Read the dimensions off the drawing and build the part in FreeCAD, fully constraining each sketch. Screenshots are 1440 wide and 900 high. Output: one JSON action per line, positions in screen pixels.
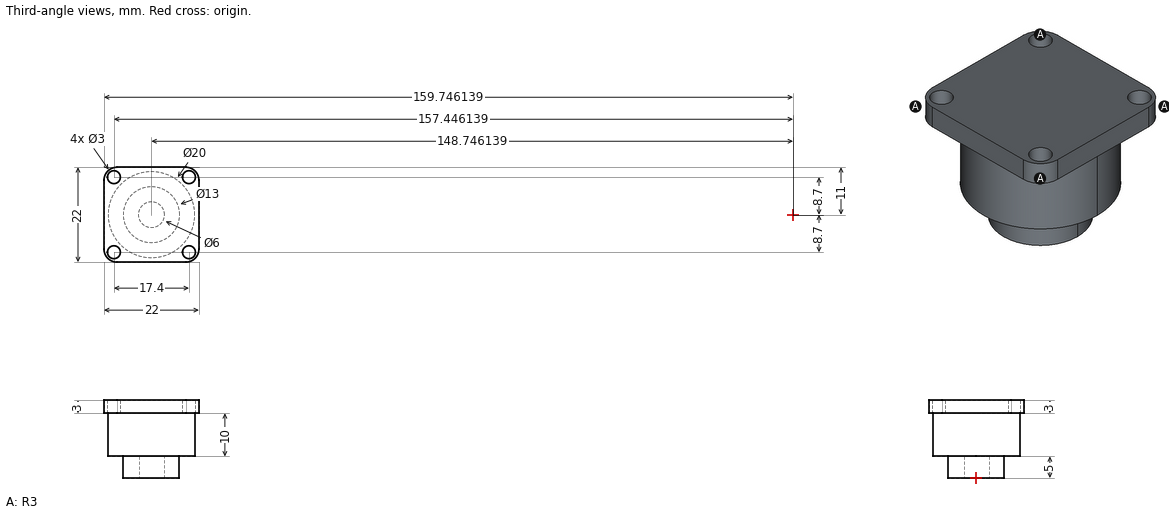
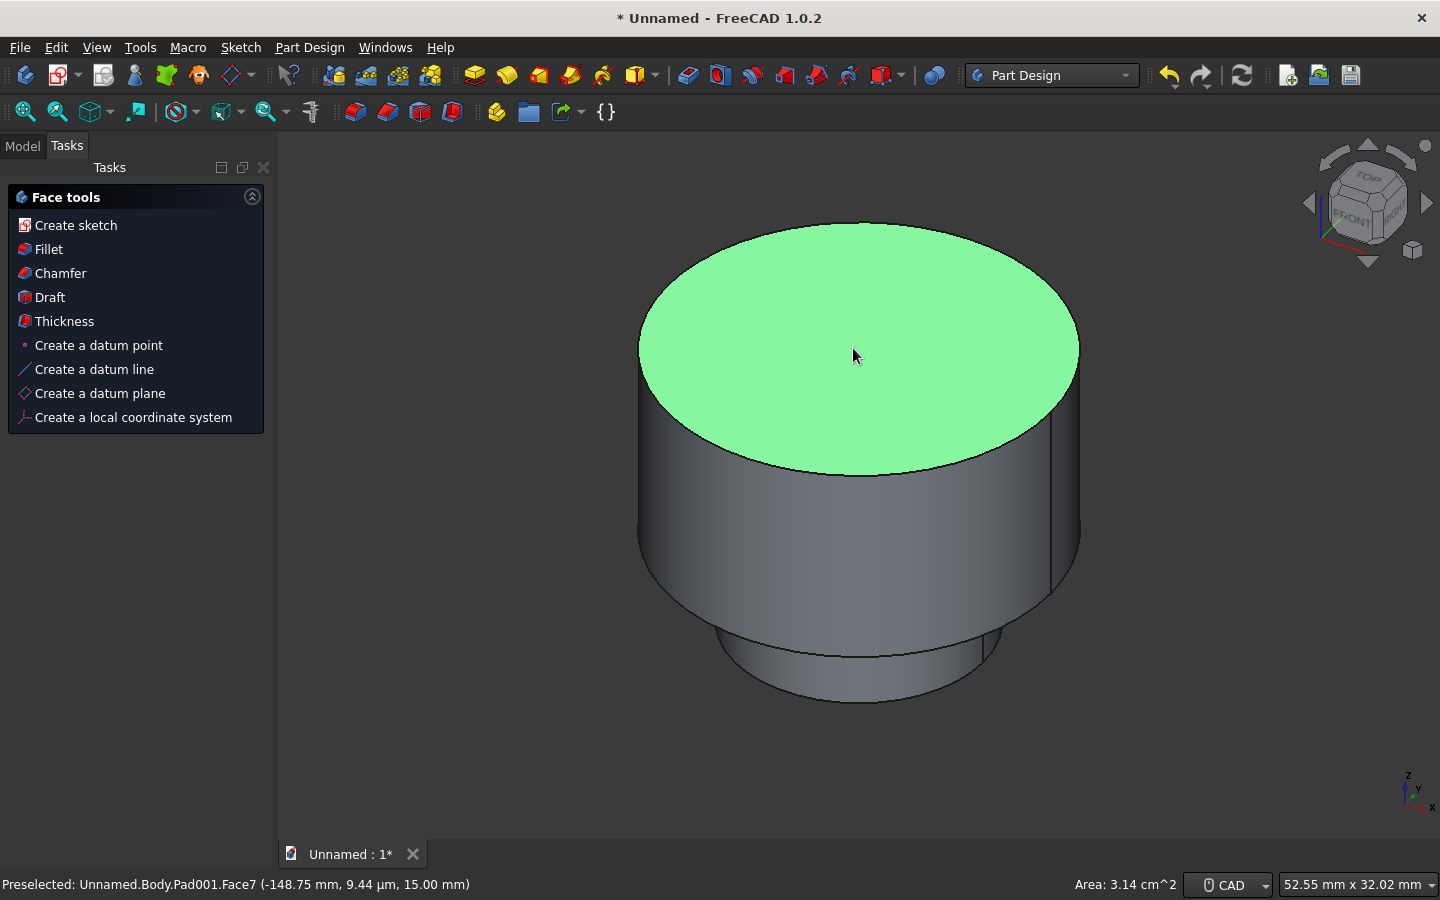
{"action": "left_click", "coordinate": [58, 76]}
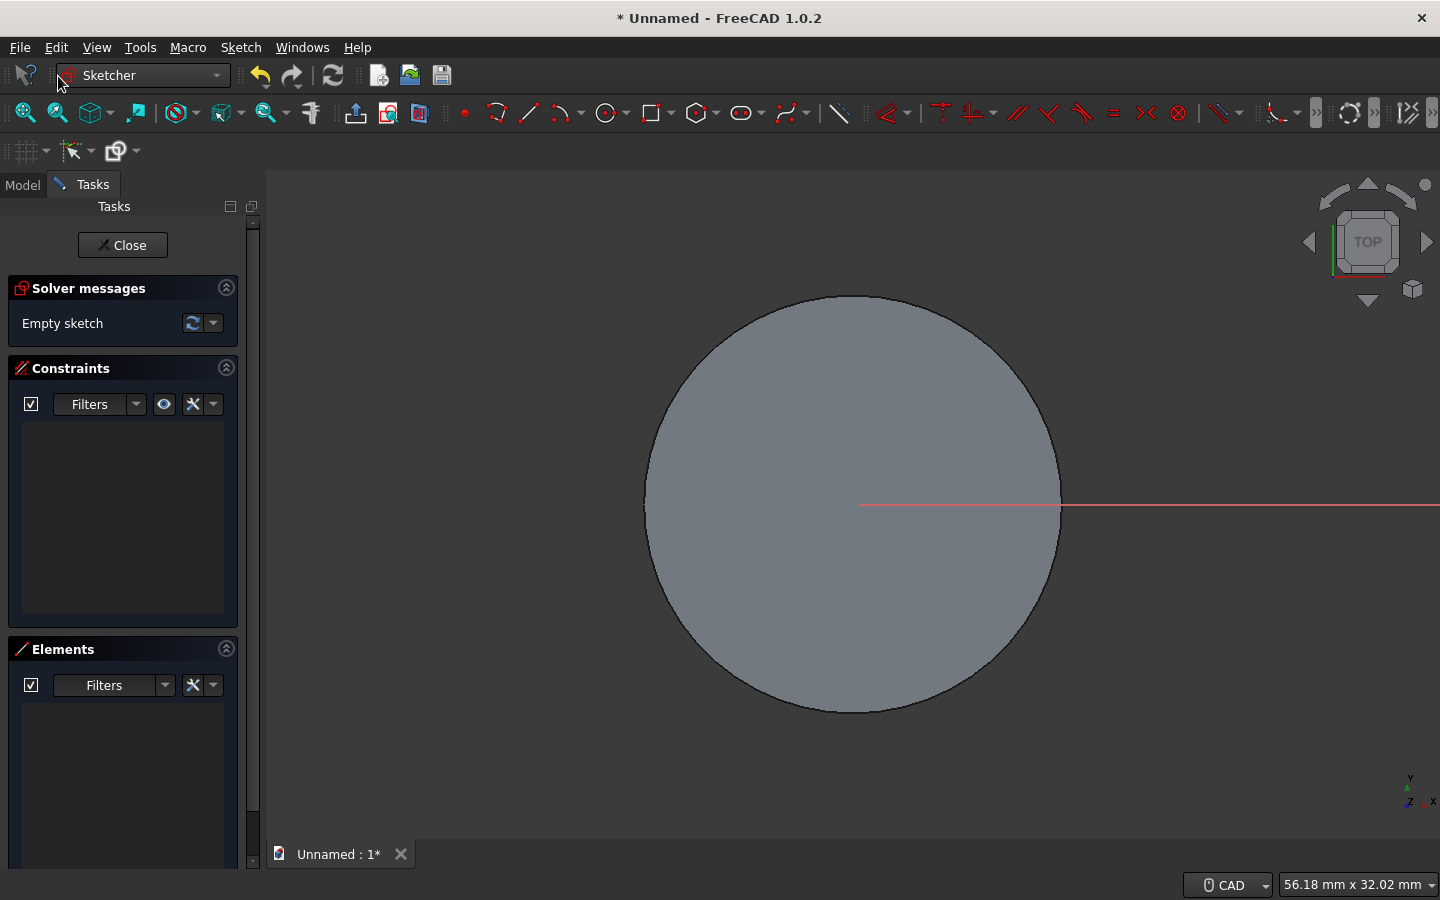
{"action": "left_click", "coordinate": [652, 114]}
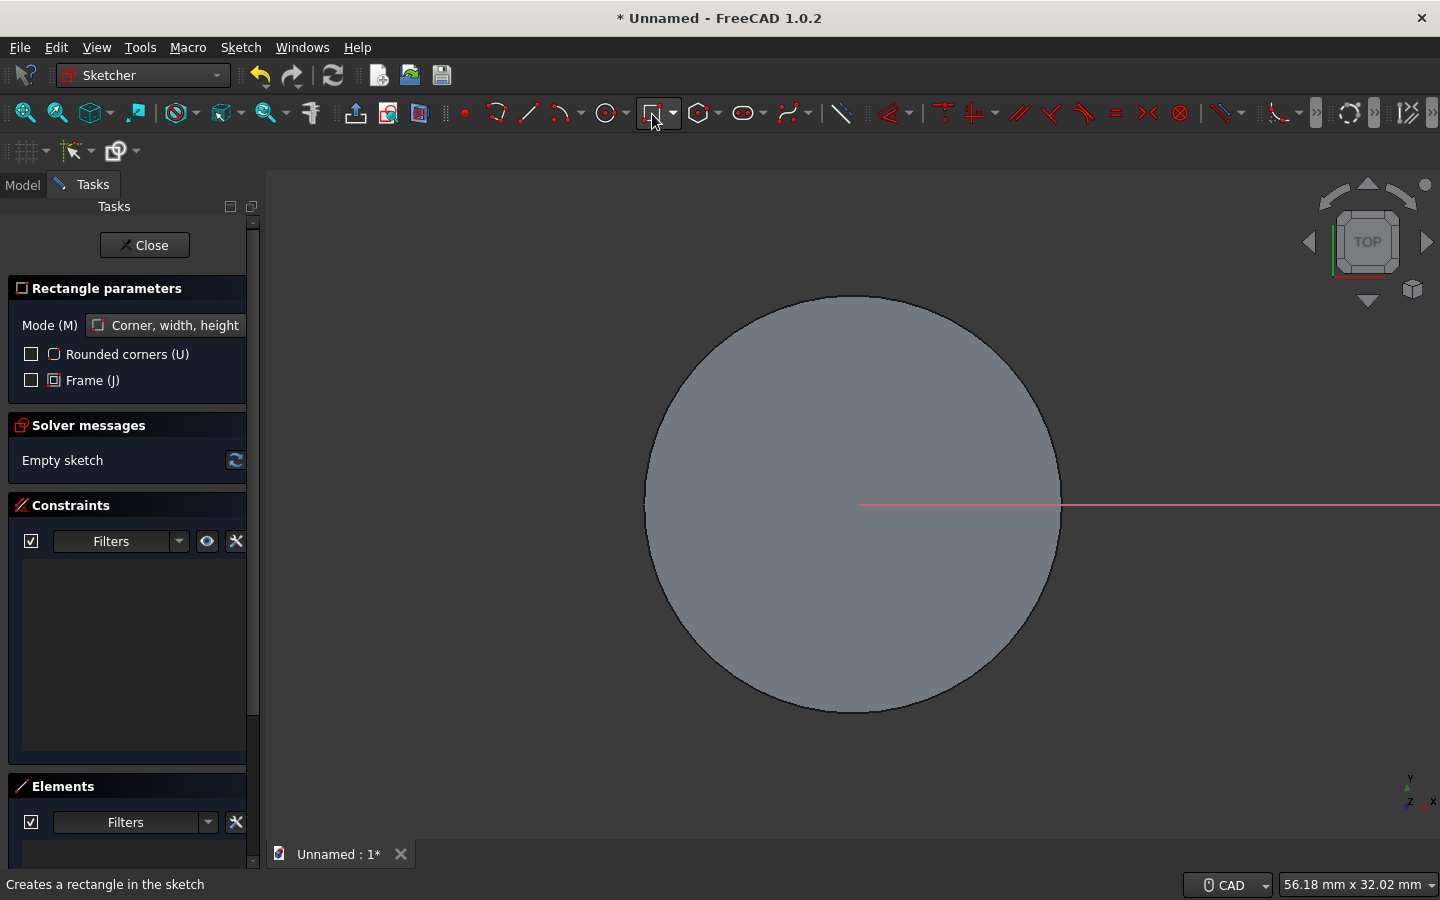
{"action": "left_click", "coordinate": [623, 275]}
{"action": "mouse_move", "coordinate": [1083, 734]}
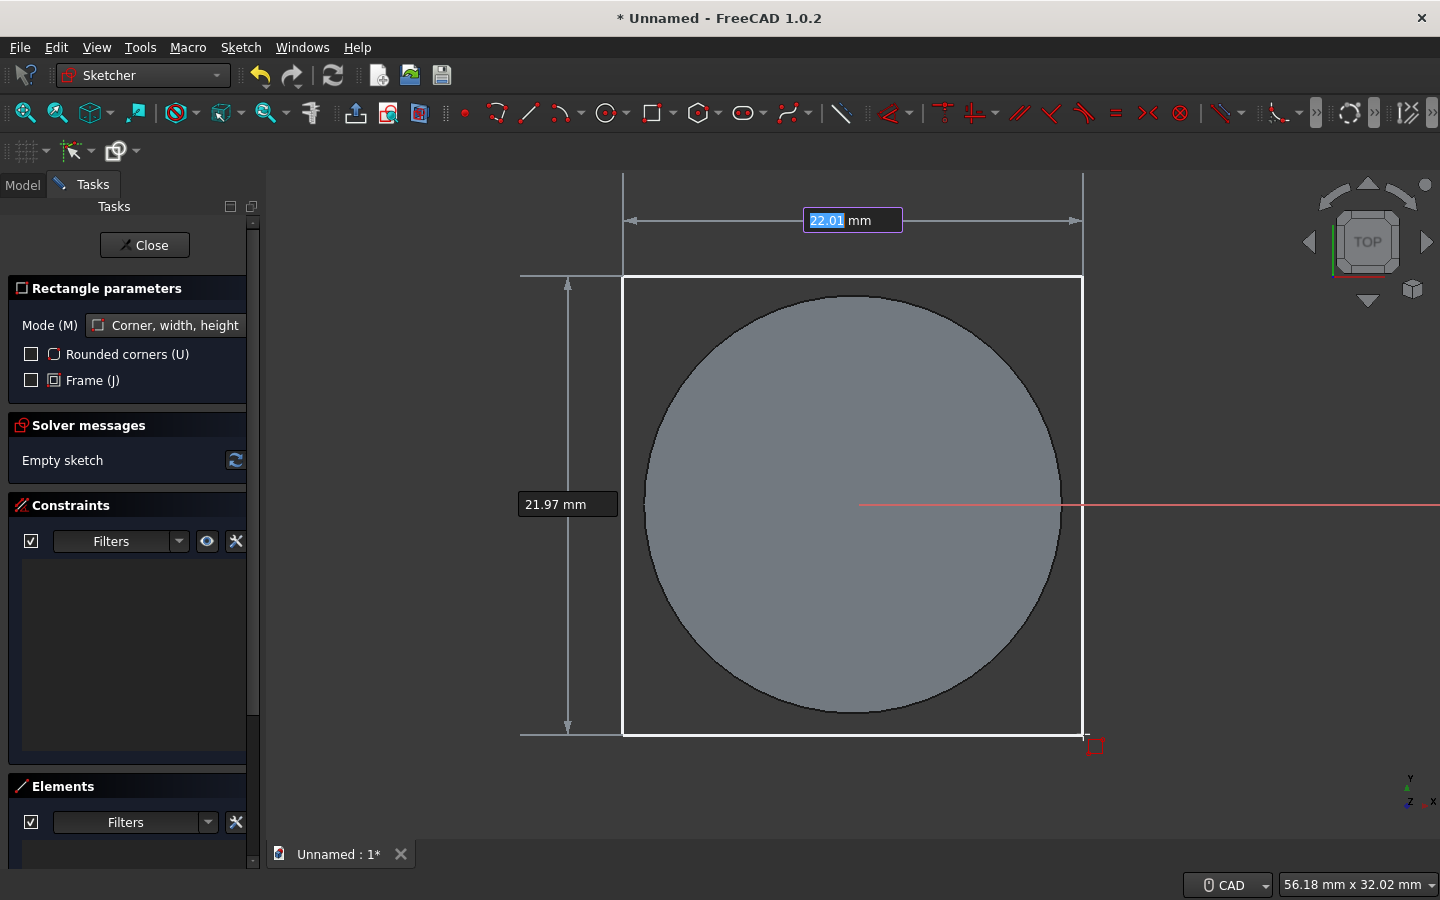
{"action": "type", "text": "22"}
{"action": "key", "text": "Tab"}
{"action": "type", "text": "22"}
{"action": "key", "text": "Return"}
{"action": "key", "text": "Escape"}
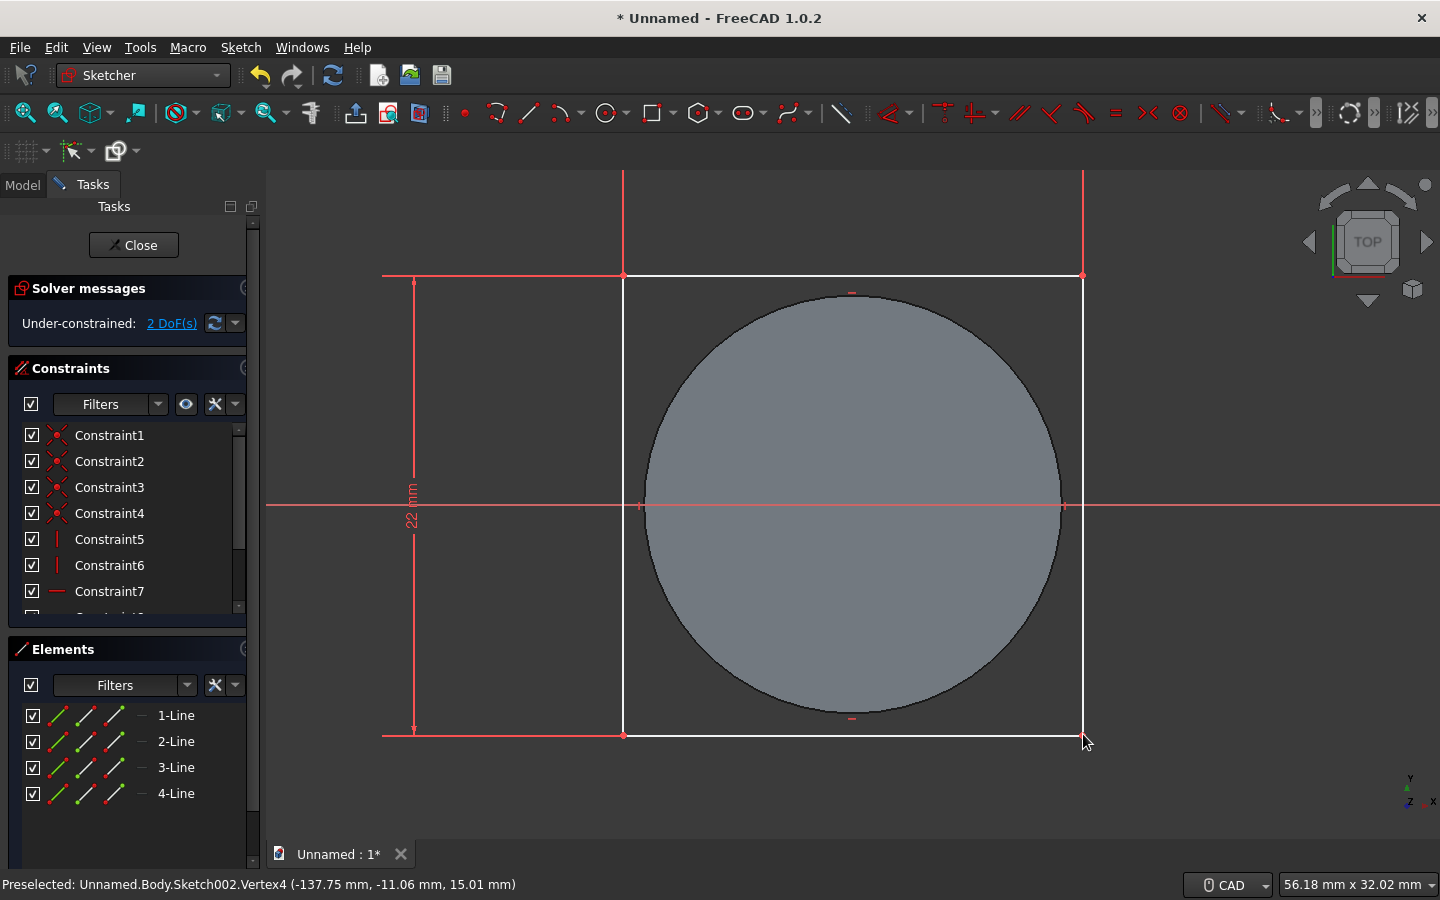
{"action": "left_click", "coordinate": [888, 114]}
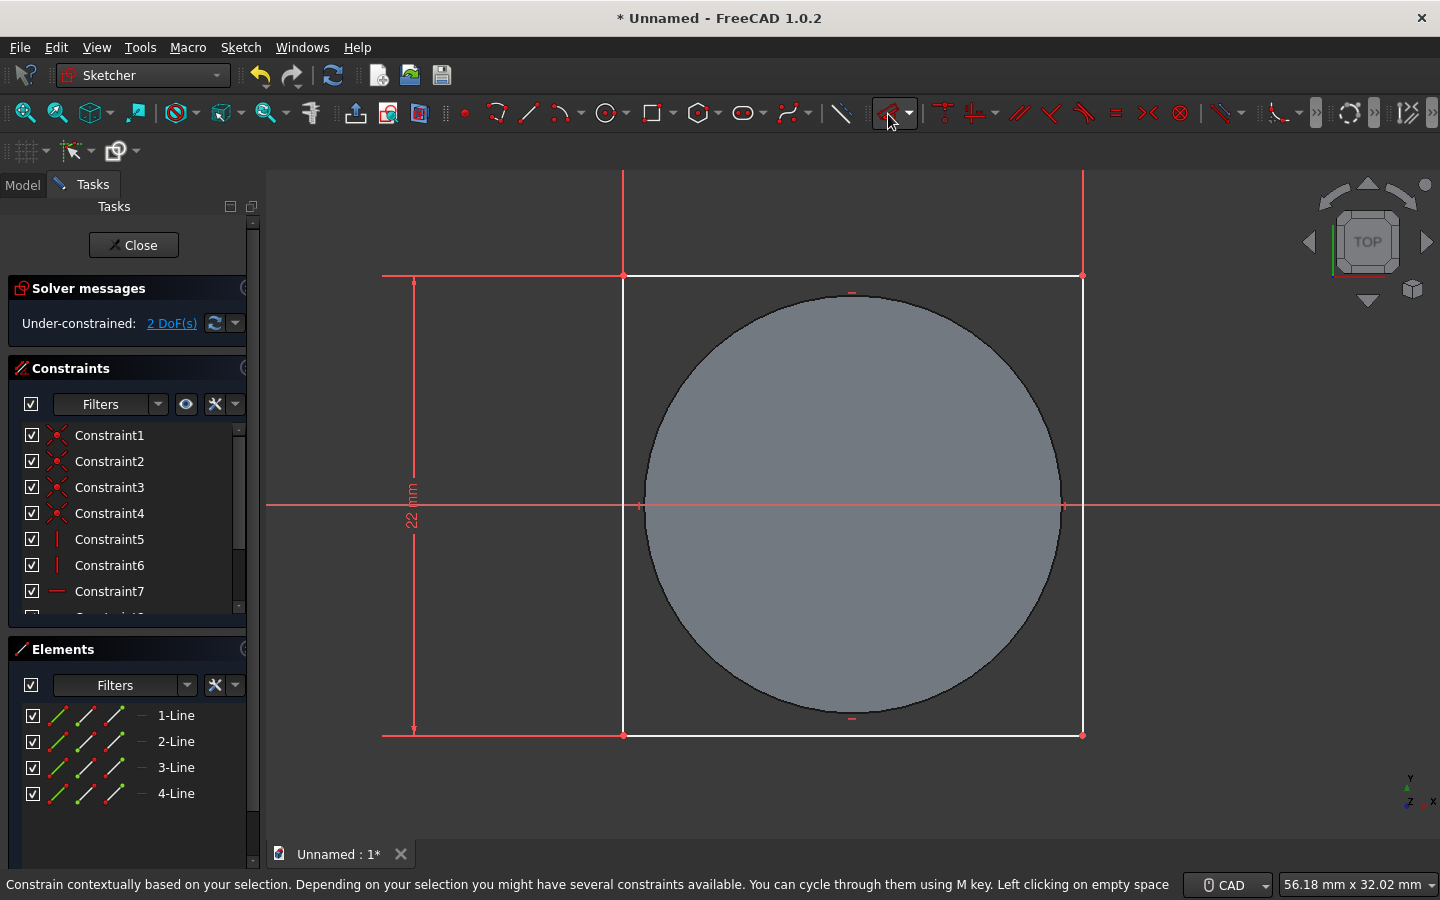
{"action": "left_click", "coordinate": [623, 276]}
{"action": "left_click", "coordinate": [589, 390]}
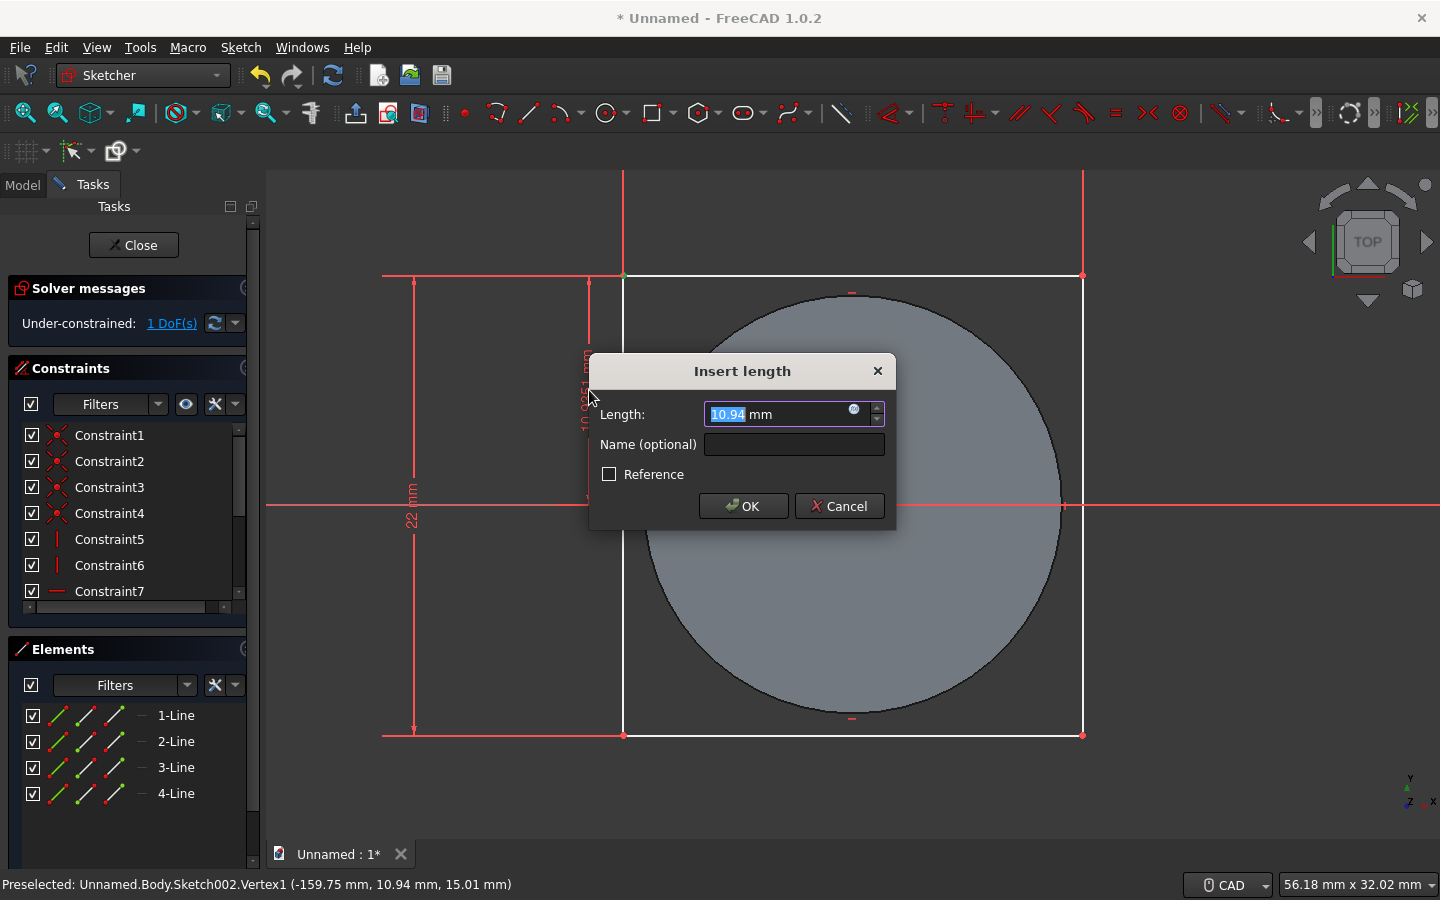
{"action": "type", "text": "11"}
{"action": "key", "text": "Return"}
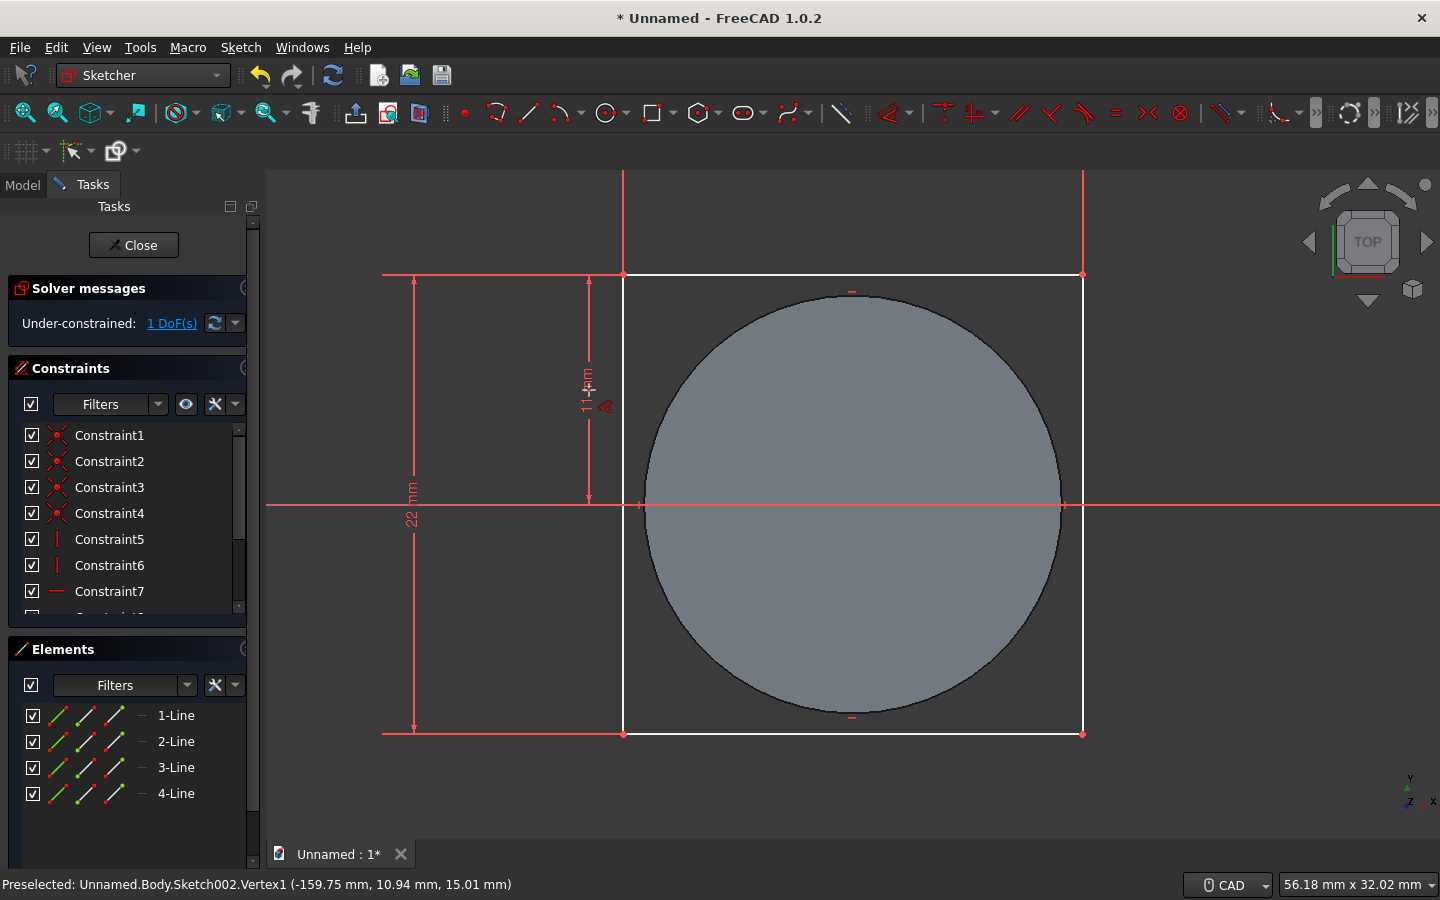
{"action": "left_click", "coordinate": [623, 275]}
{"action": "left_click", "coordinate": [949, 241]}